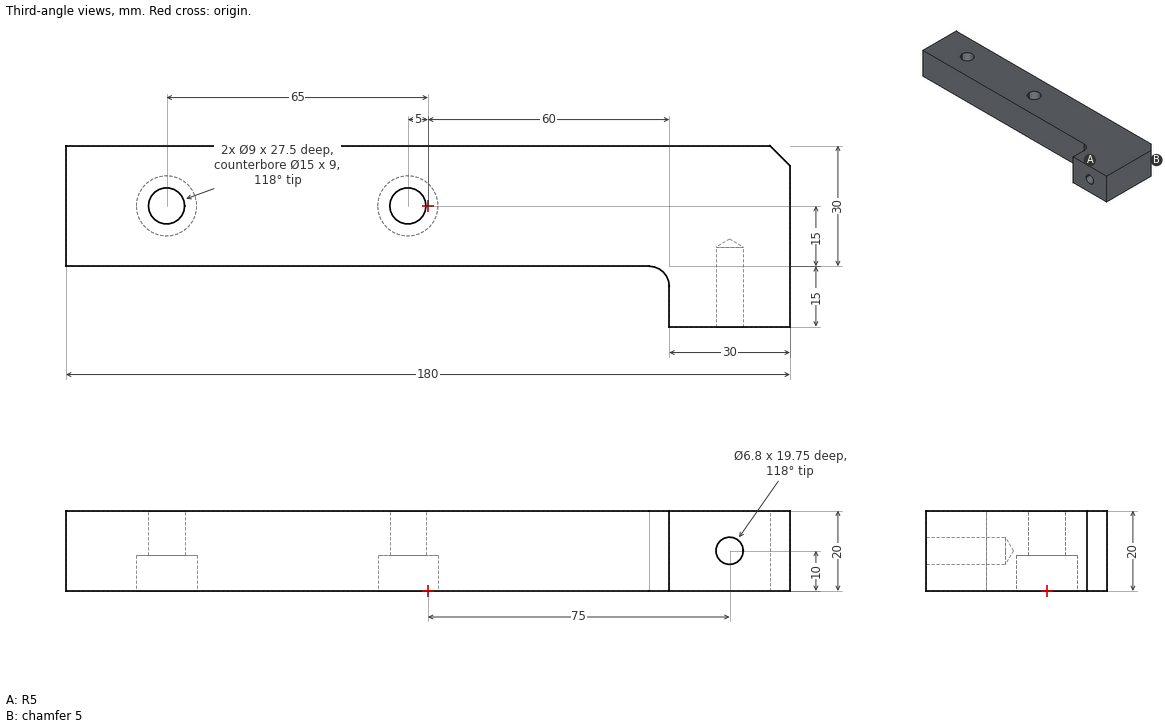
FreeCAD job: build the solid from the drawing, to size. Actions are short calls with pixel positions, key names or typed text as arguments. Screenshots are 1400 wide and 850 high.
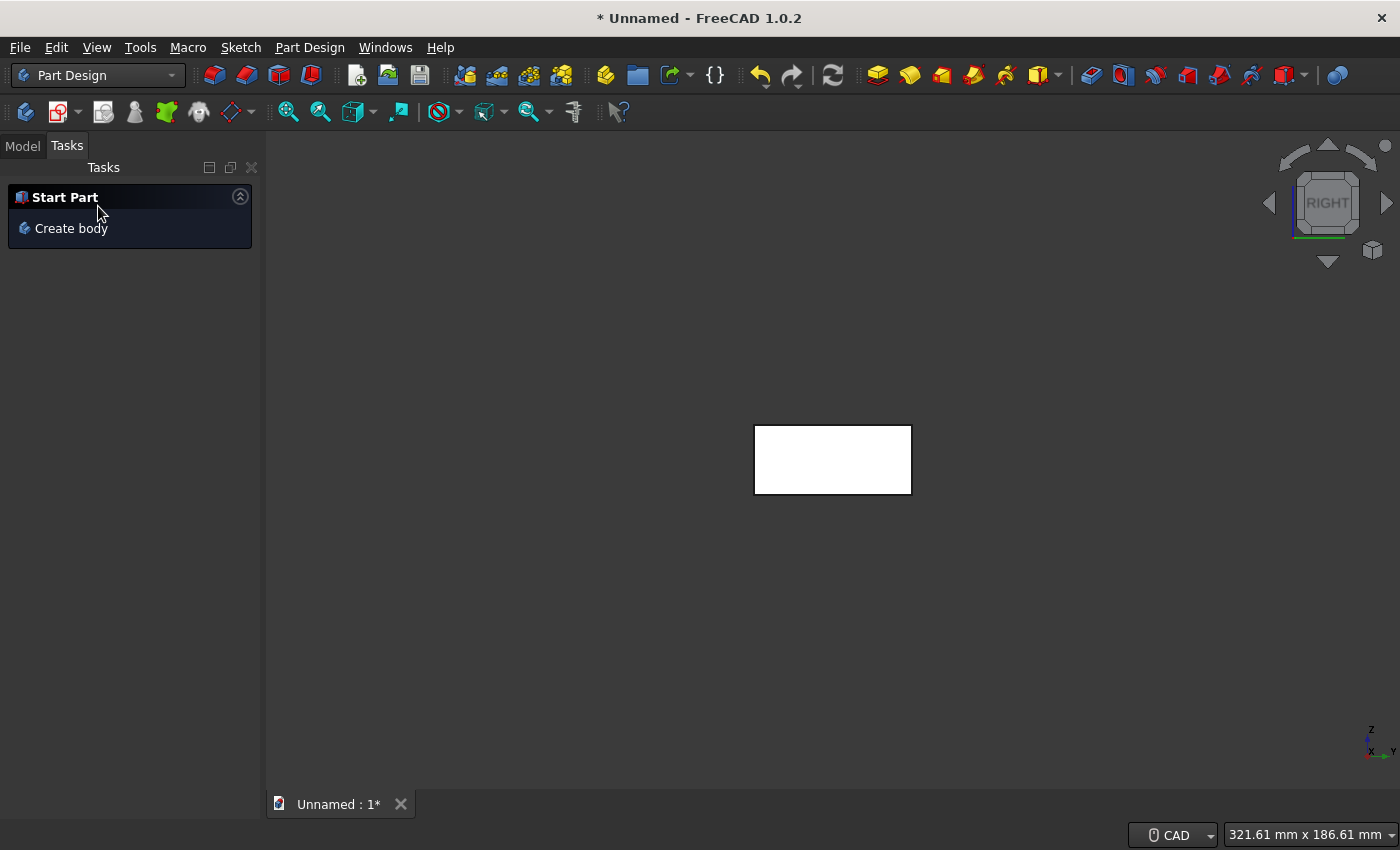
click(290, 112)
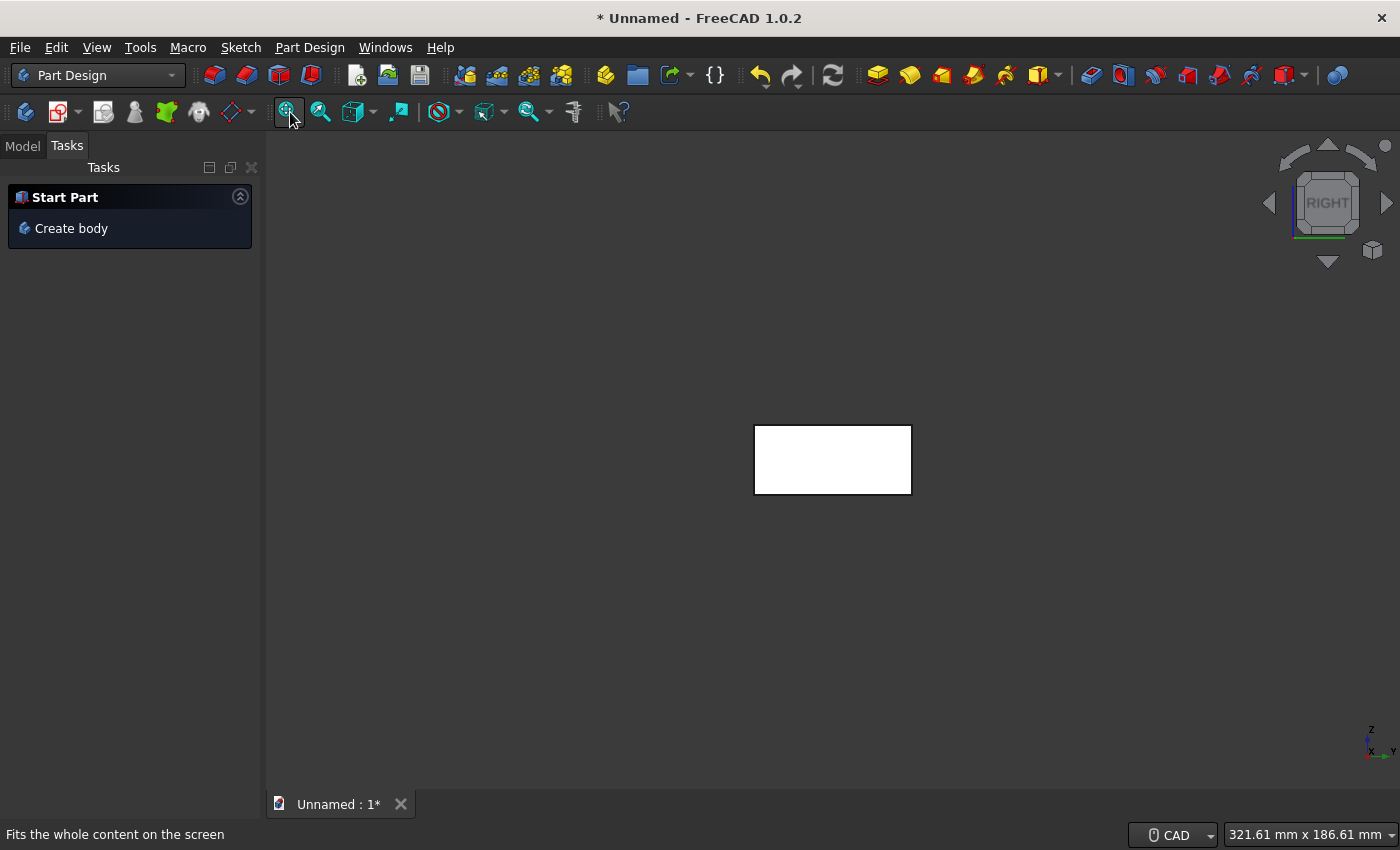
click(912, 459)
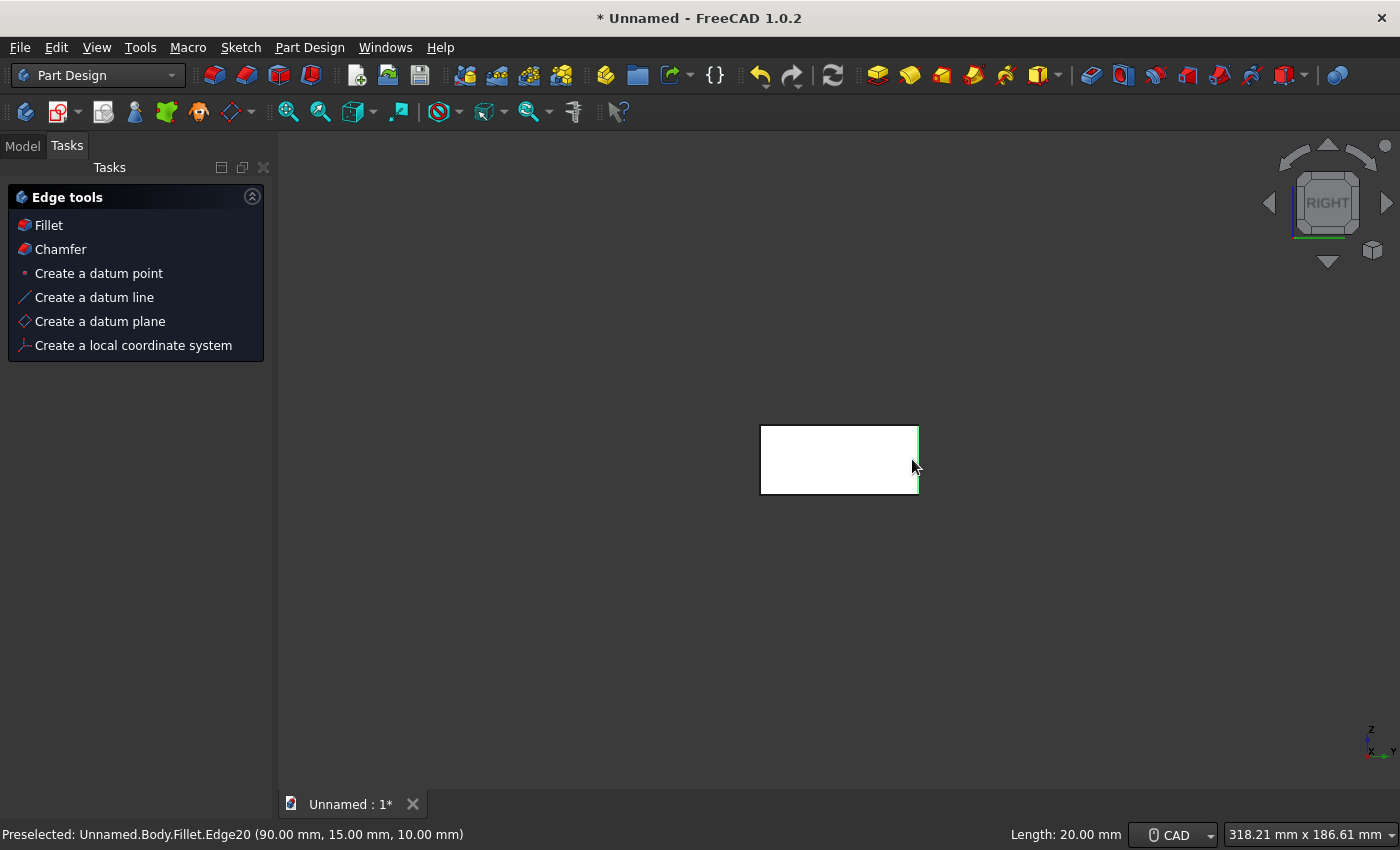
click(248, 76)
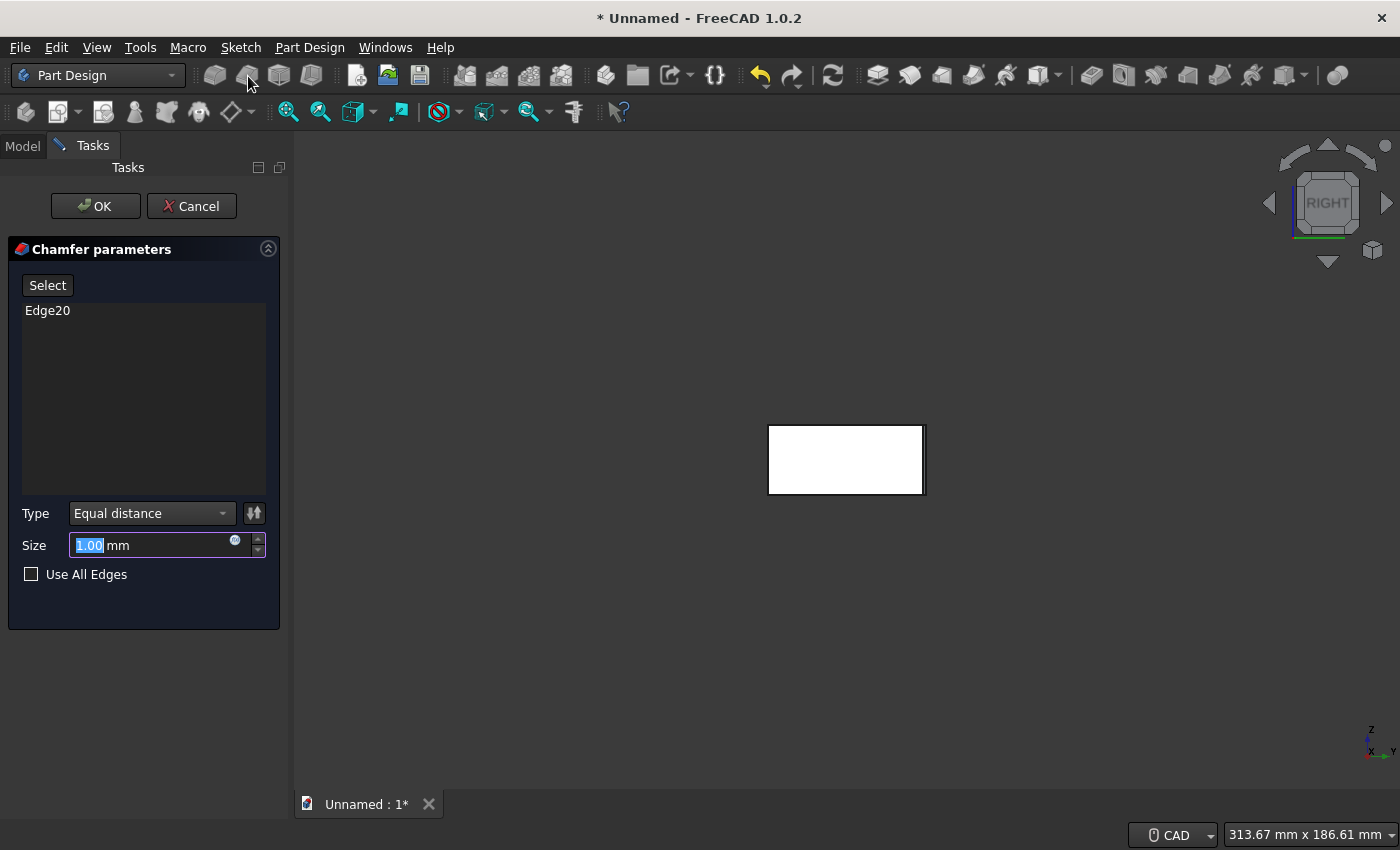
text(5)
key(Tab)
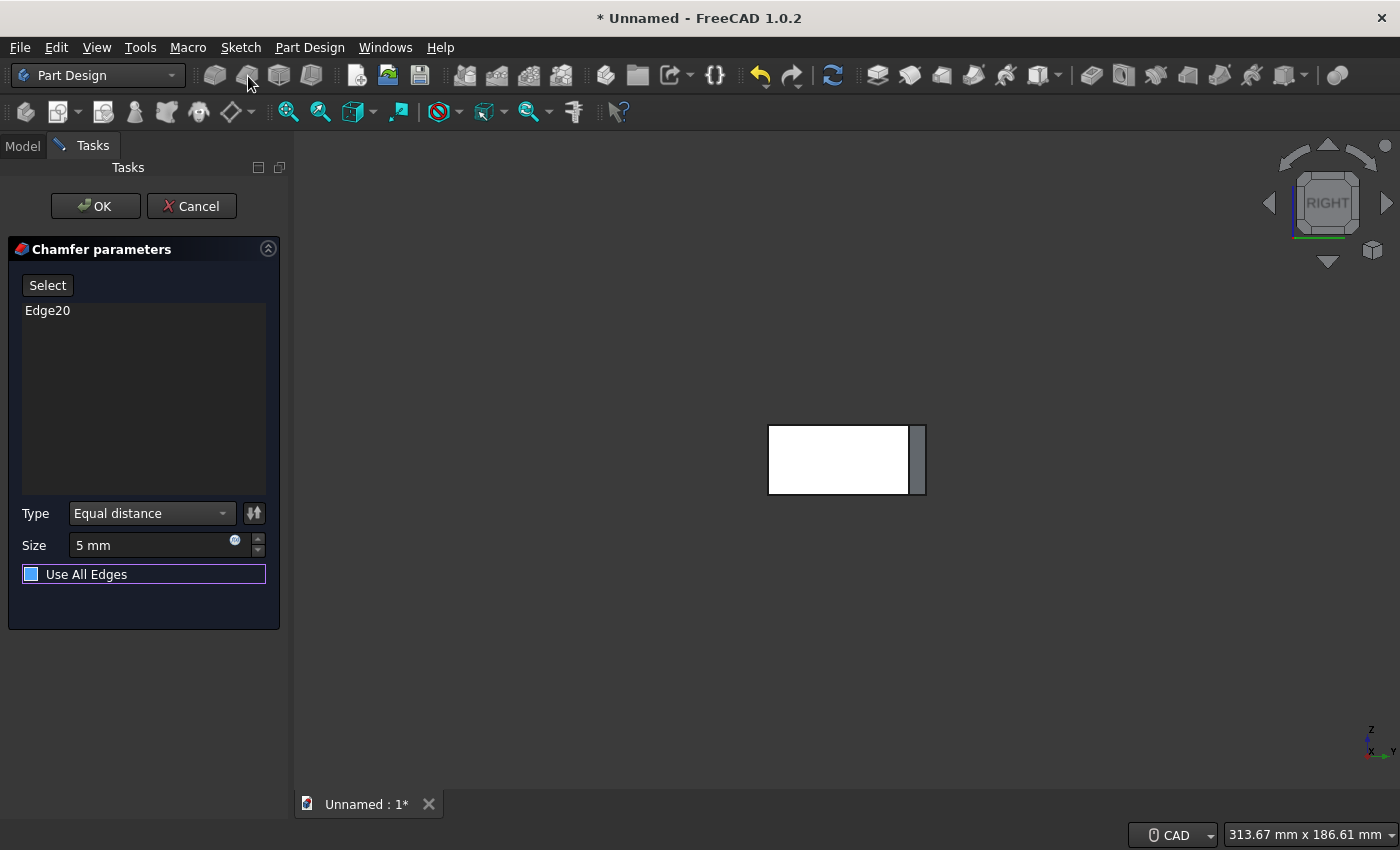
click(96, 206)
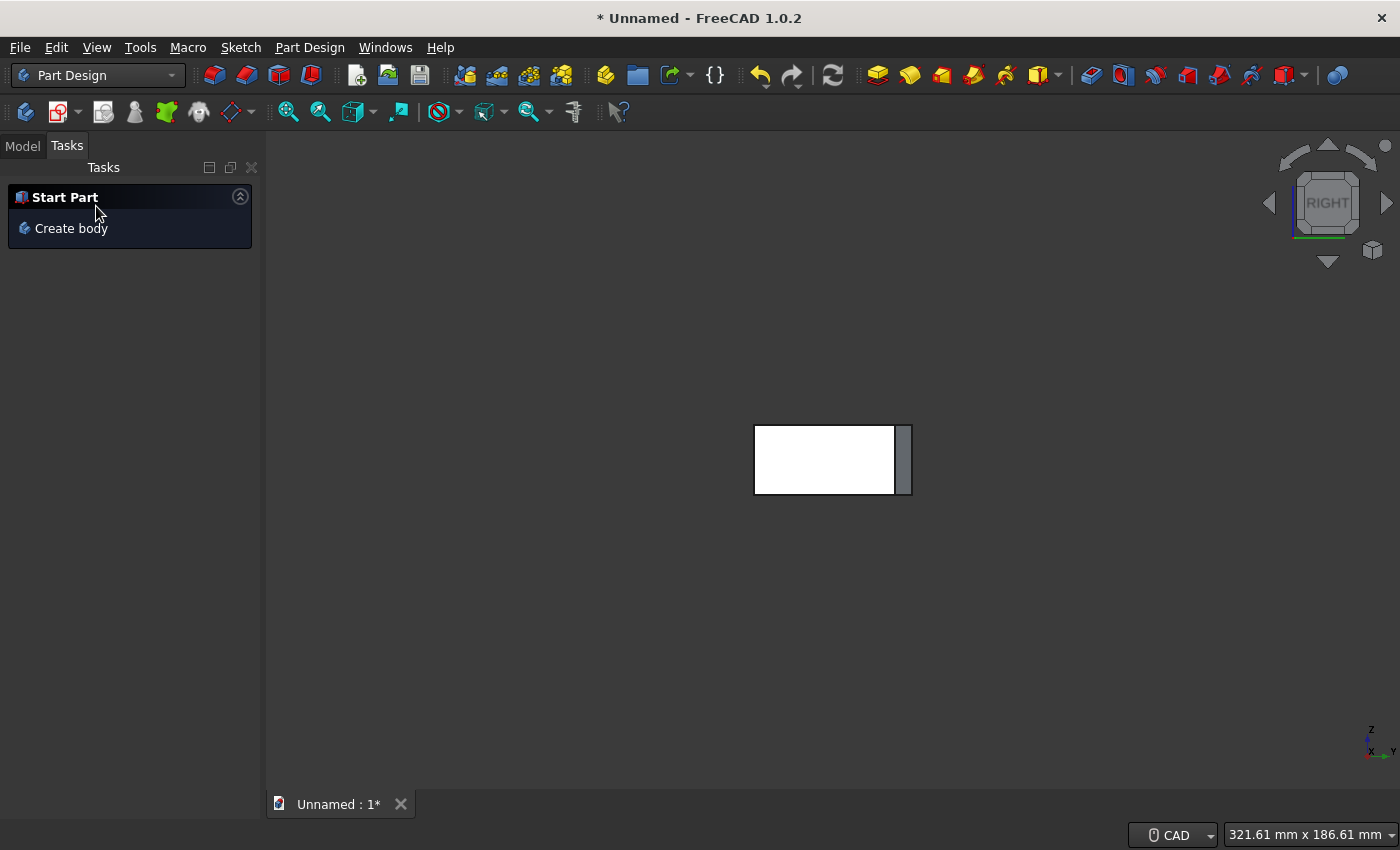
click(290, 112)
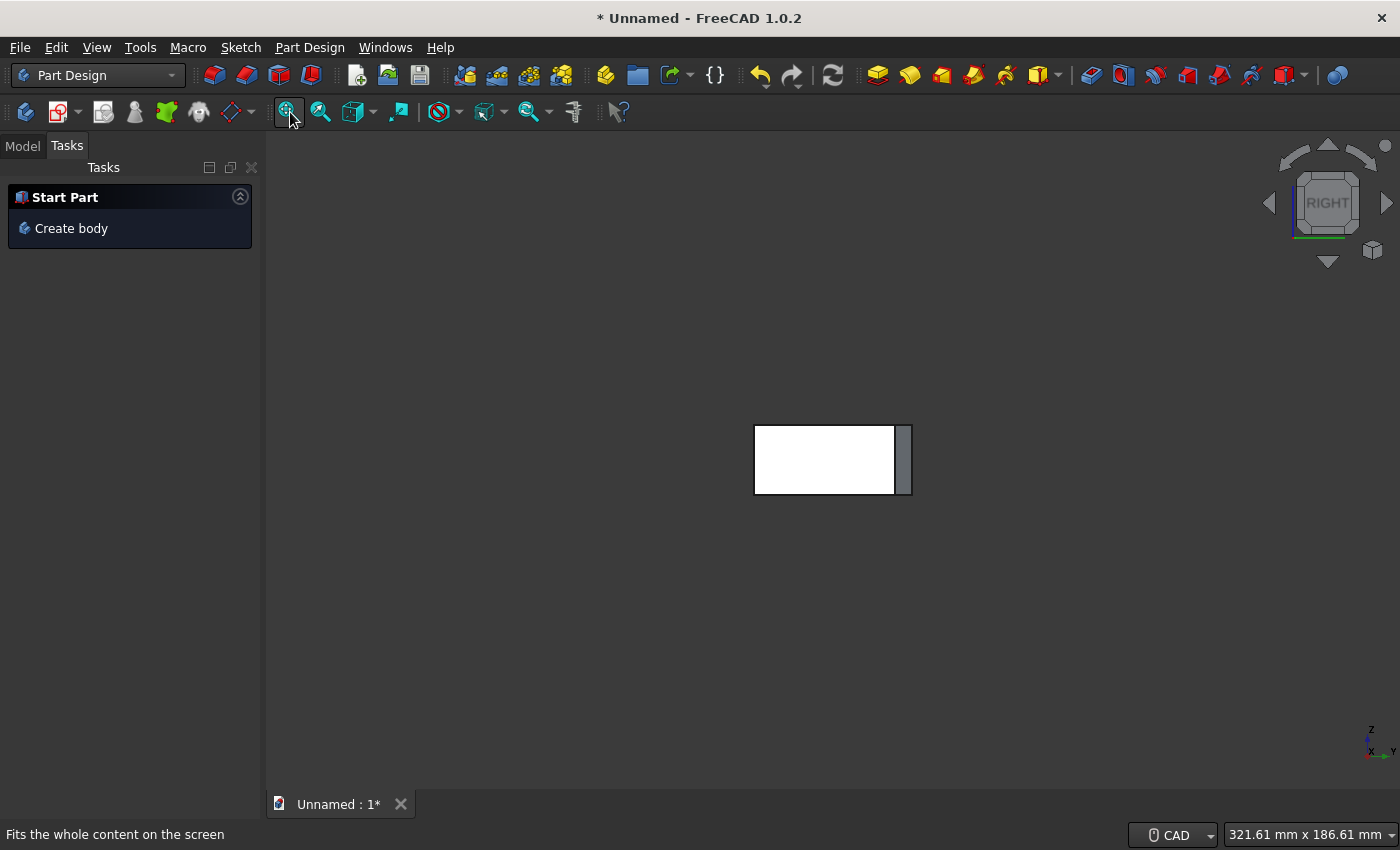
key(0)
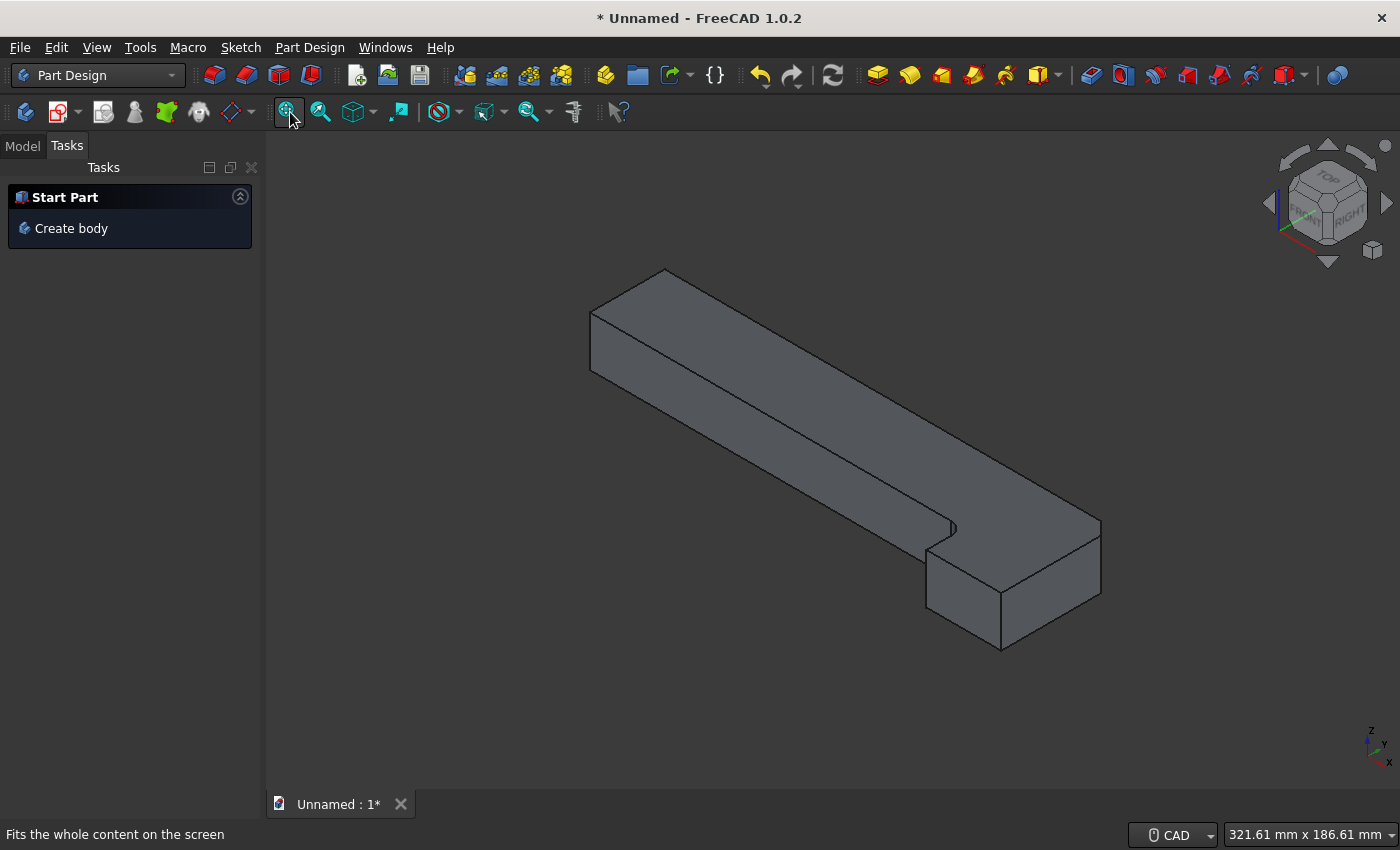
click(975, 606)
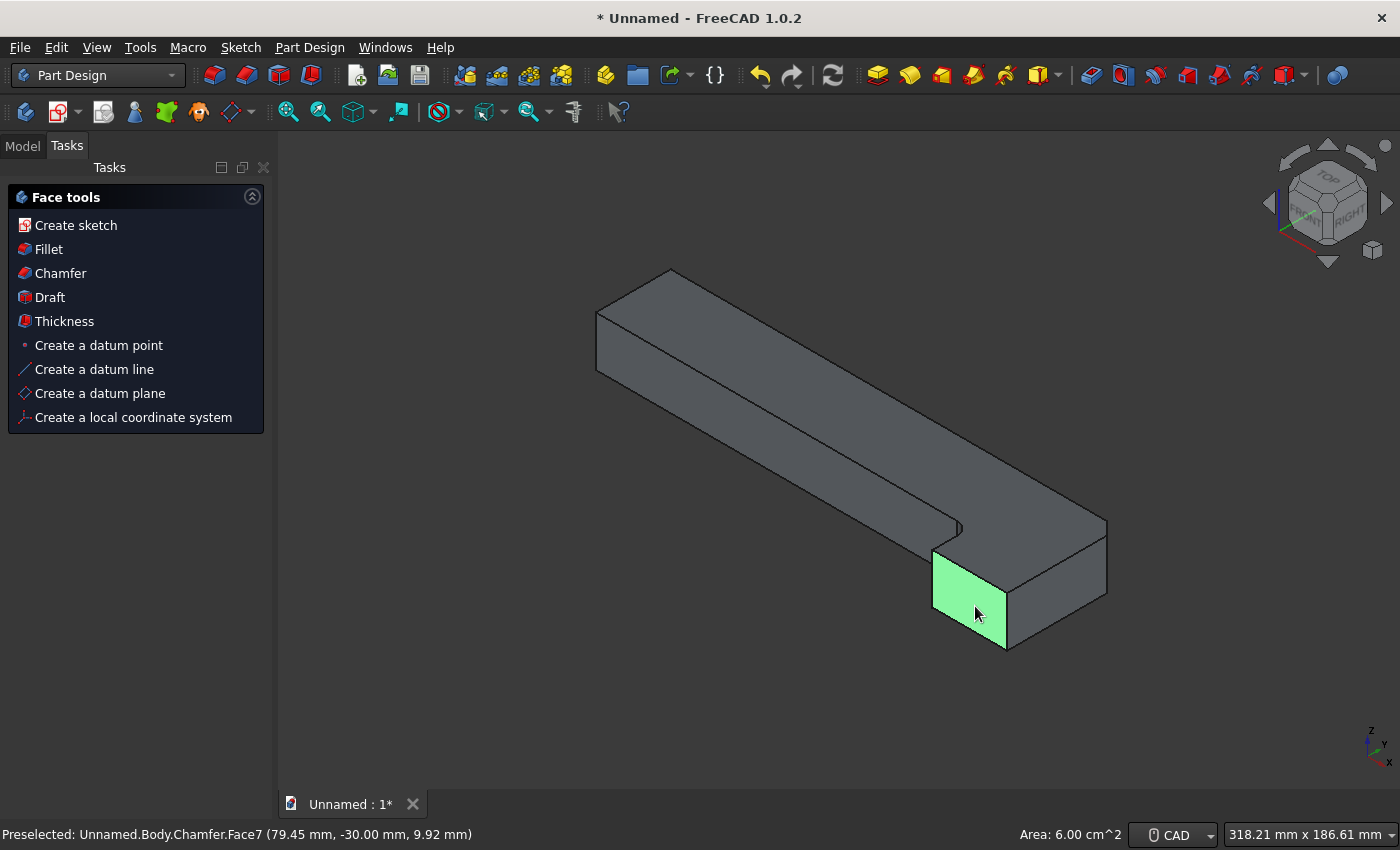
click(58, 112)